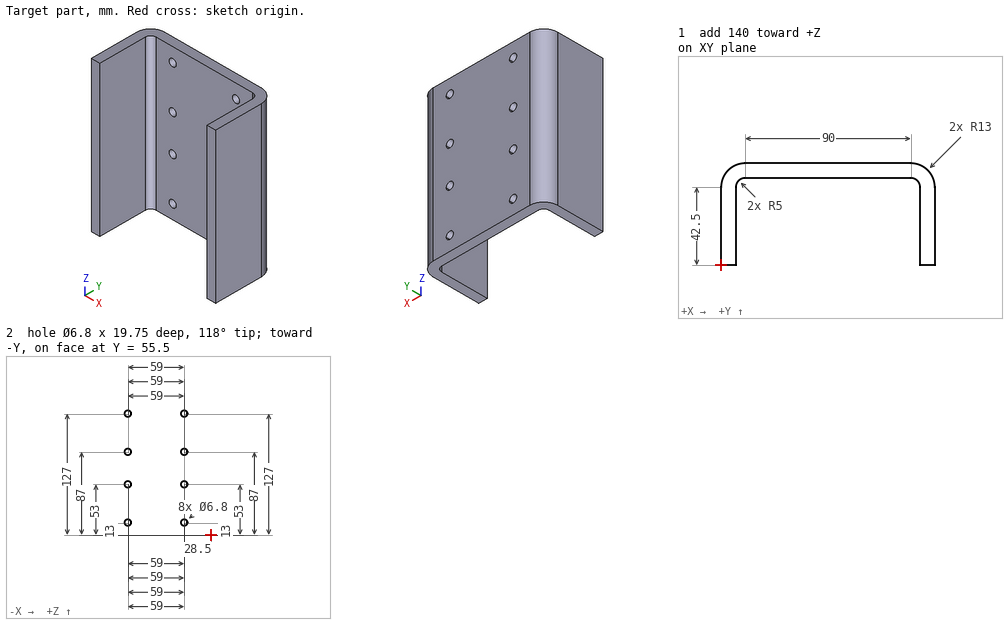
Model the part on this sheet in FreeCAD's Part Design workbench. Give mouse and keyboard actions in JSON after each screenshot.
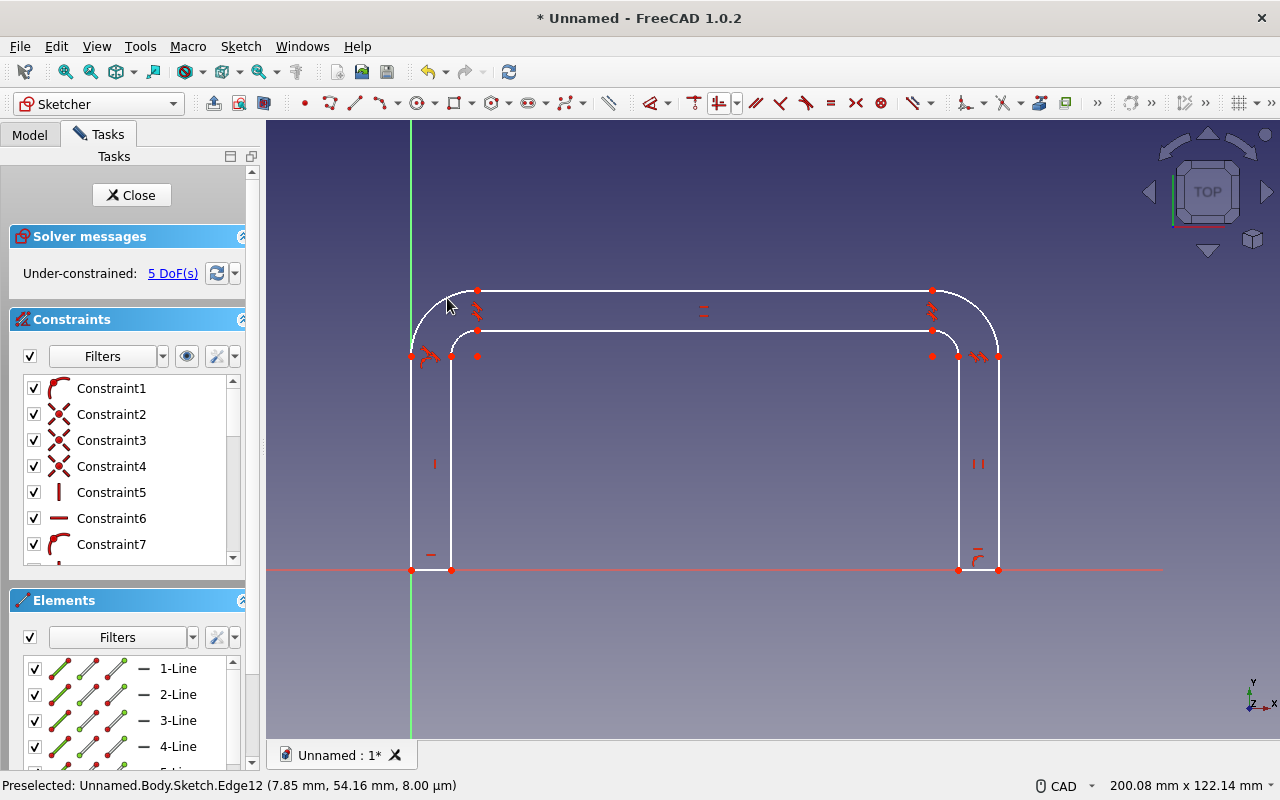
{"action": "left_click", "coordinate": [465, 333]}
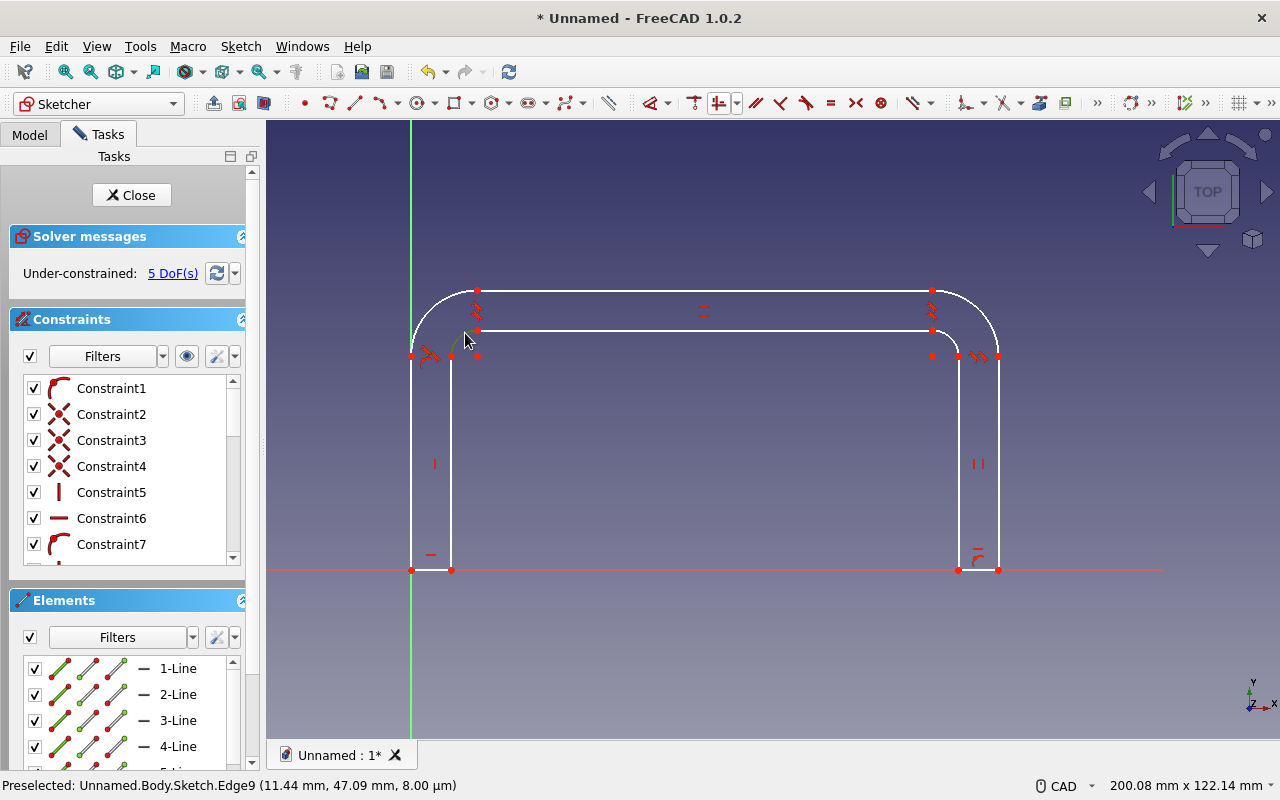
{"action": "left_click", "coordinate": [956, 345]}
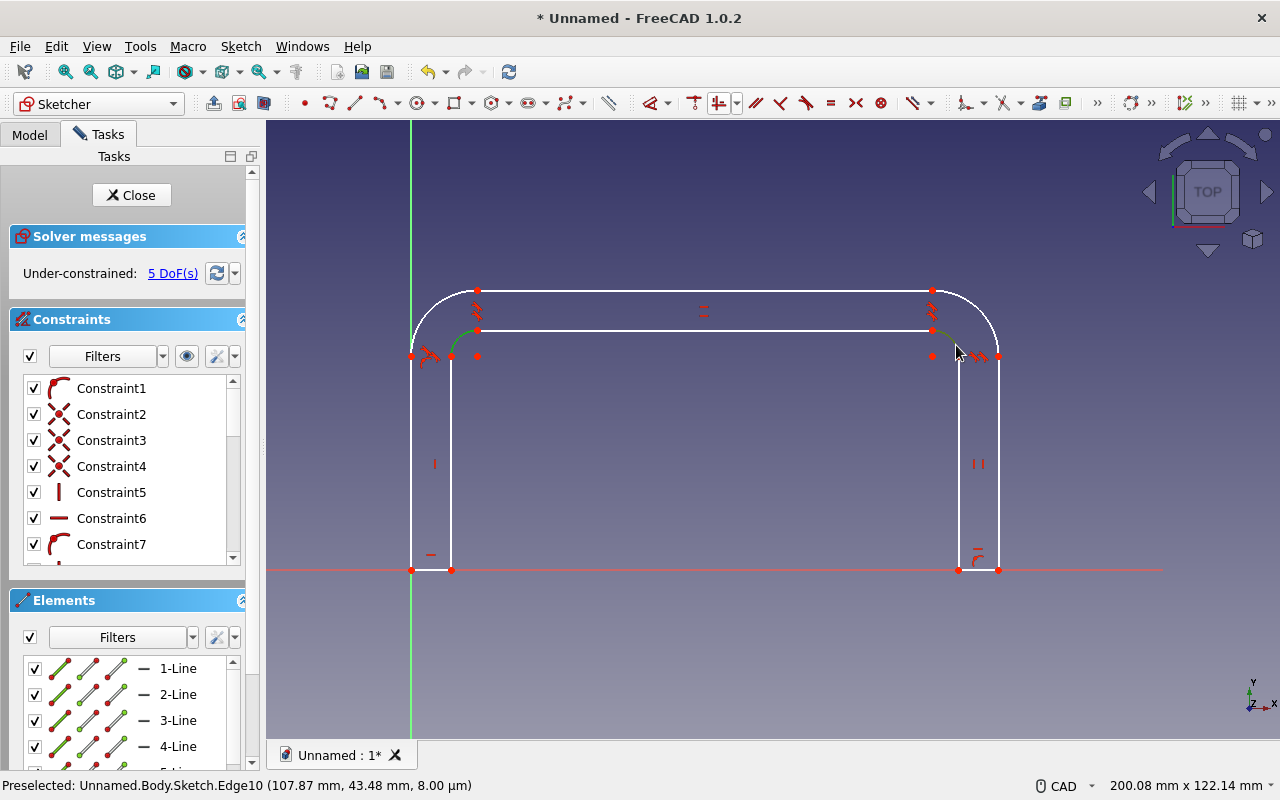
{"action": "left_click", "coordinate": [831, 104]}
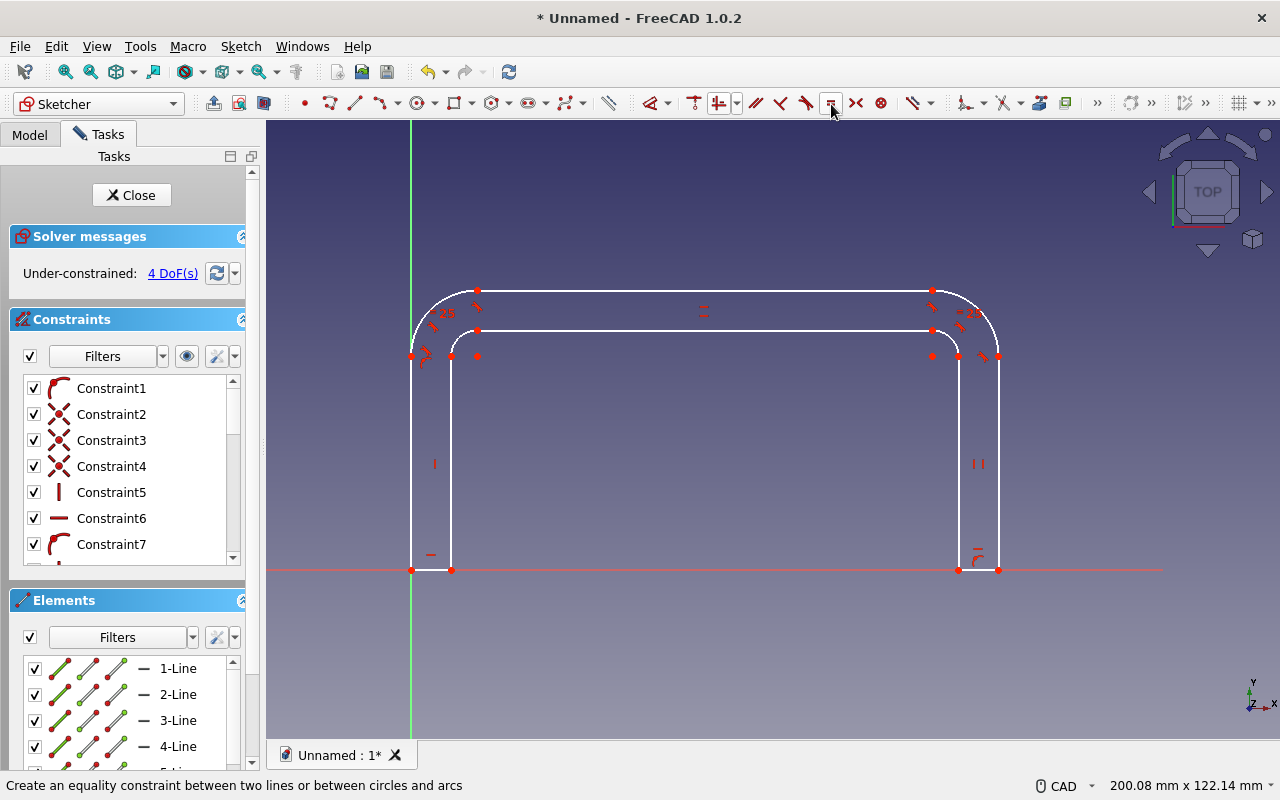
{"action": "key", "text": "d"}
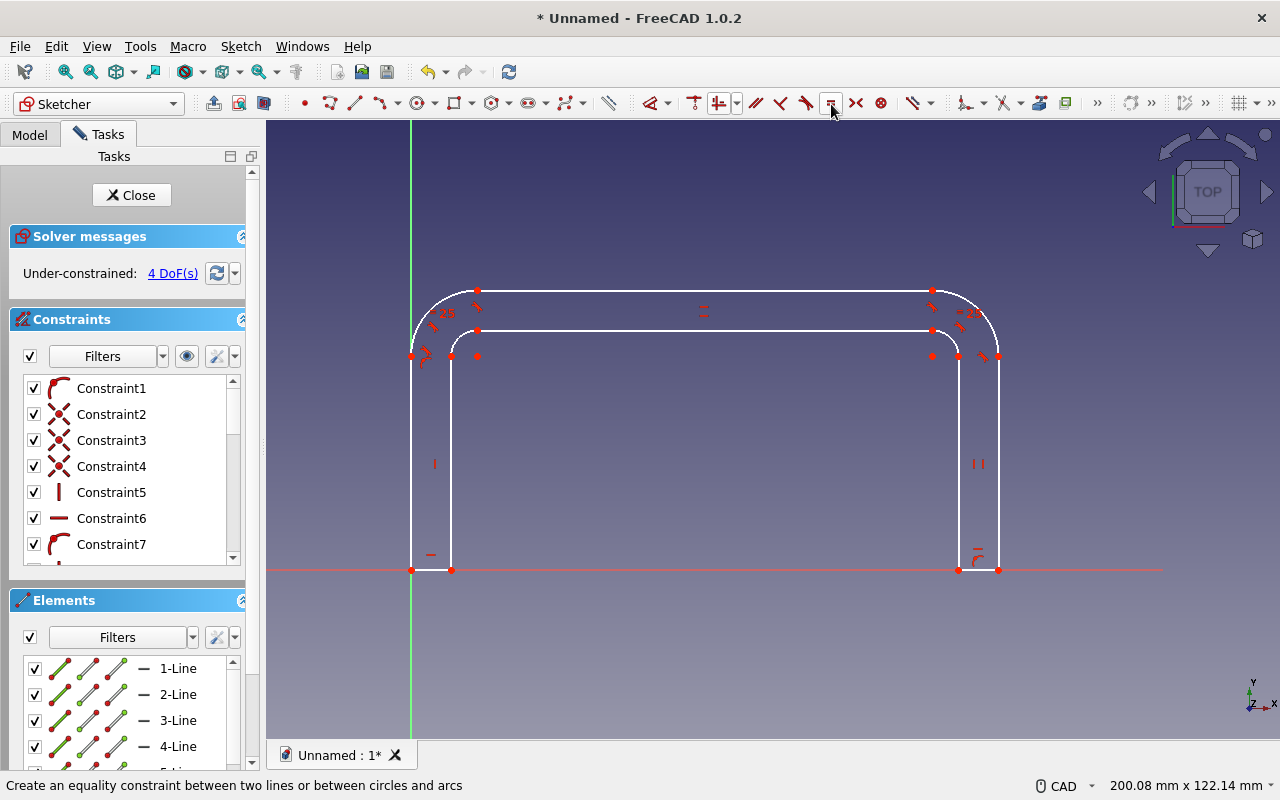
{"action": "scroll", "coordinate": [465, 333], "scroll_direction": "up", "scroll_amount": 3}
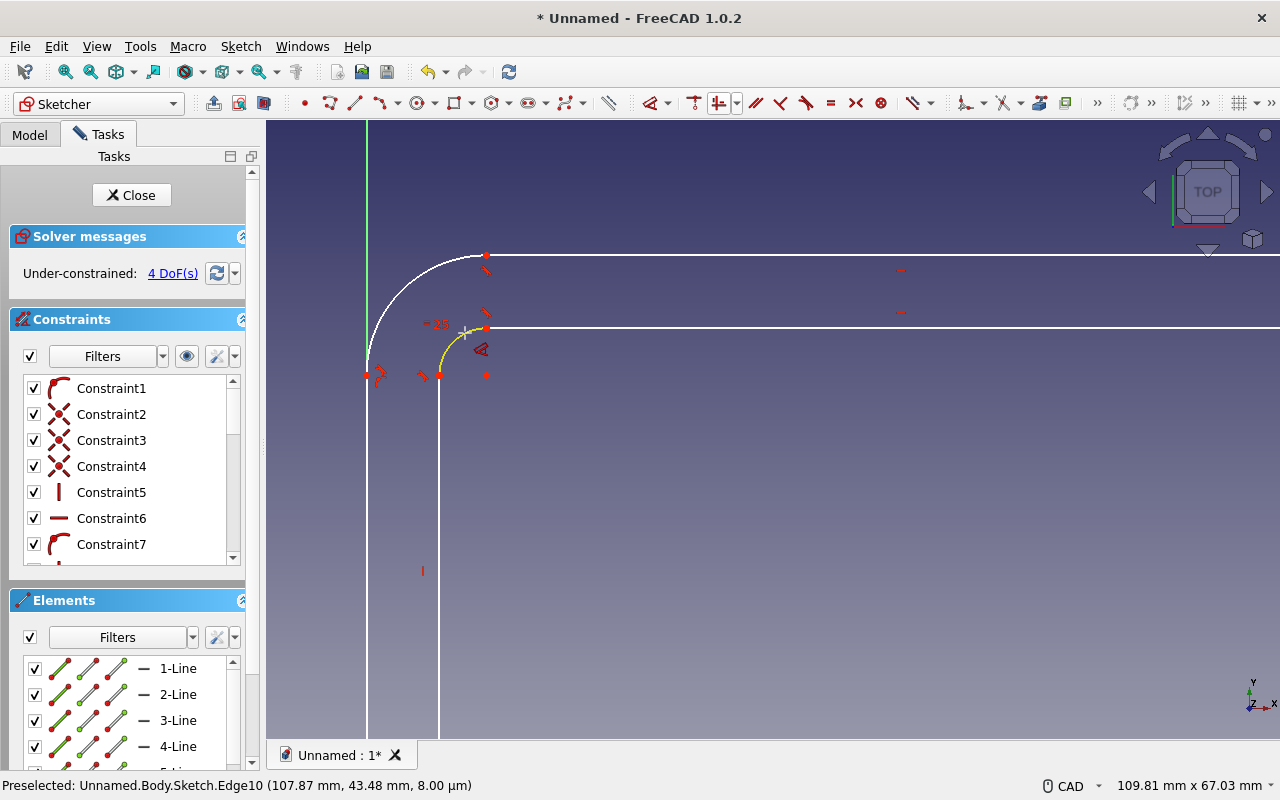
{"action": "left_click", "coordinate": [465, 333]}
{"action": "left_click", "coordinate": [450, 305]}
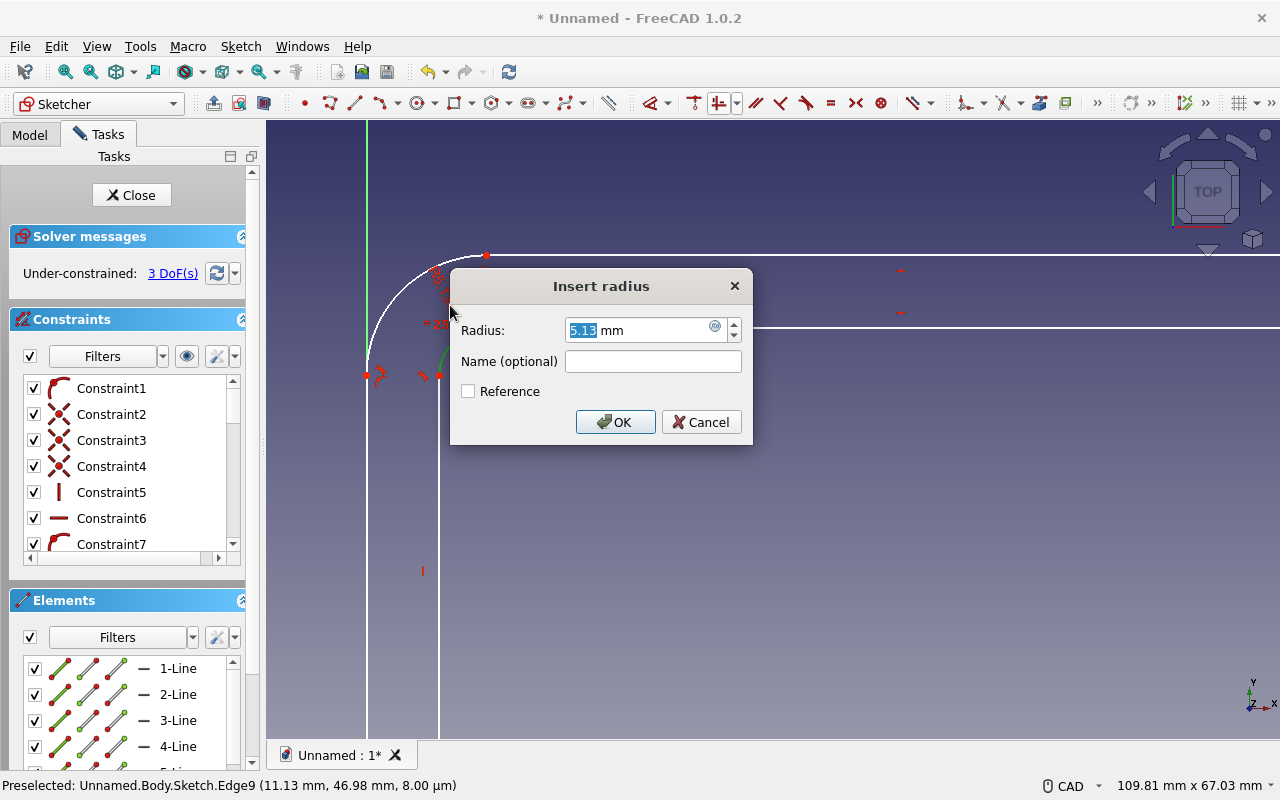
{"action": "type", "text": "5"}
{"action": "key", "text": "Return"}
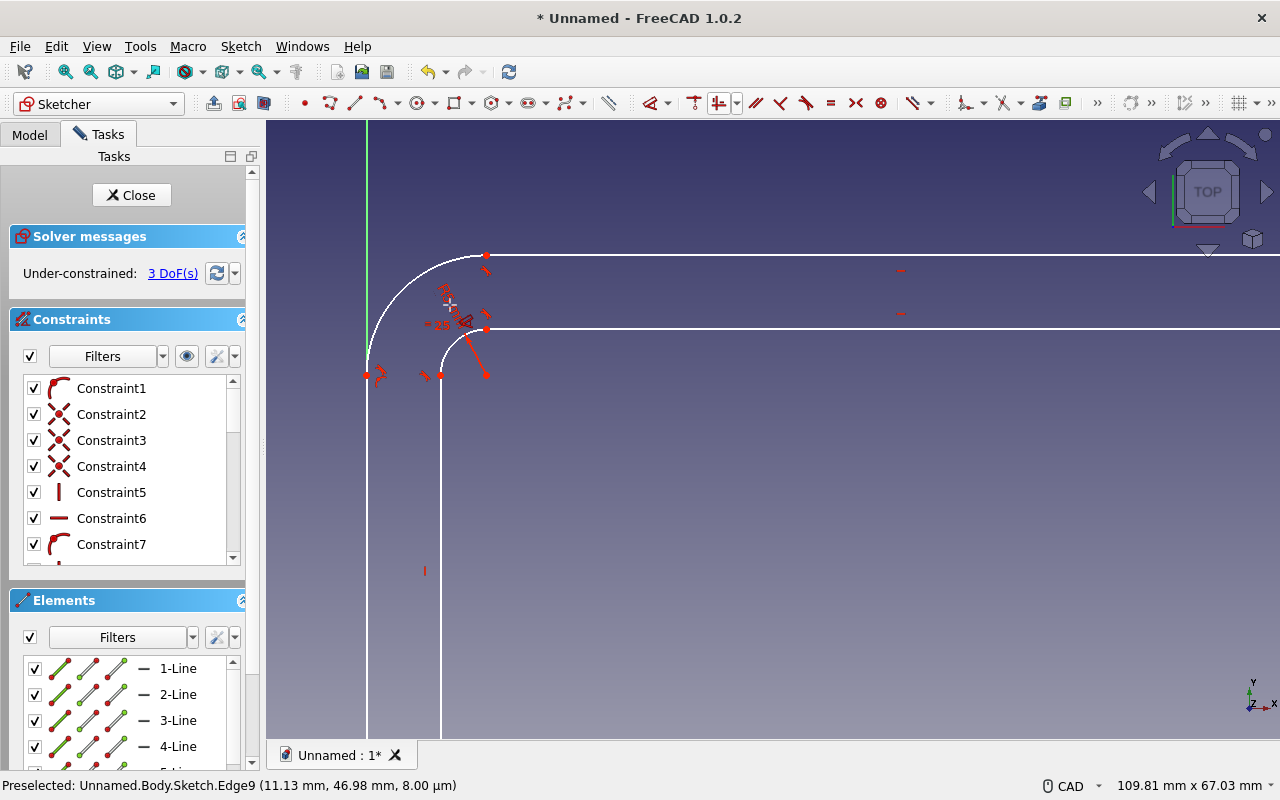
{"action": "scroll", "coordinate": [464, 333], "scroll_direction": "down", "scroll_amount": 3}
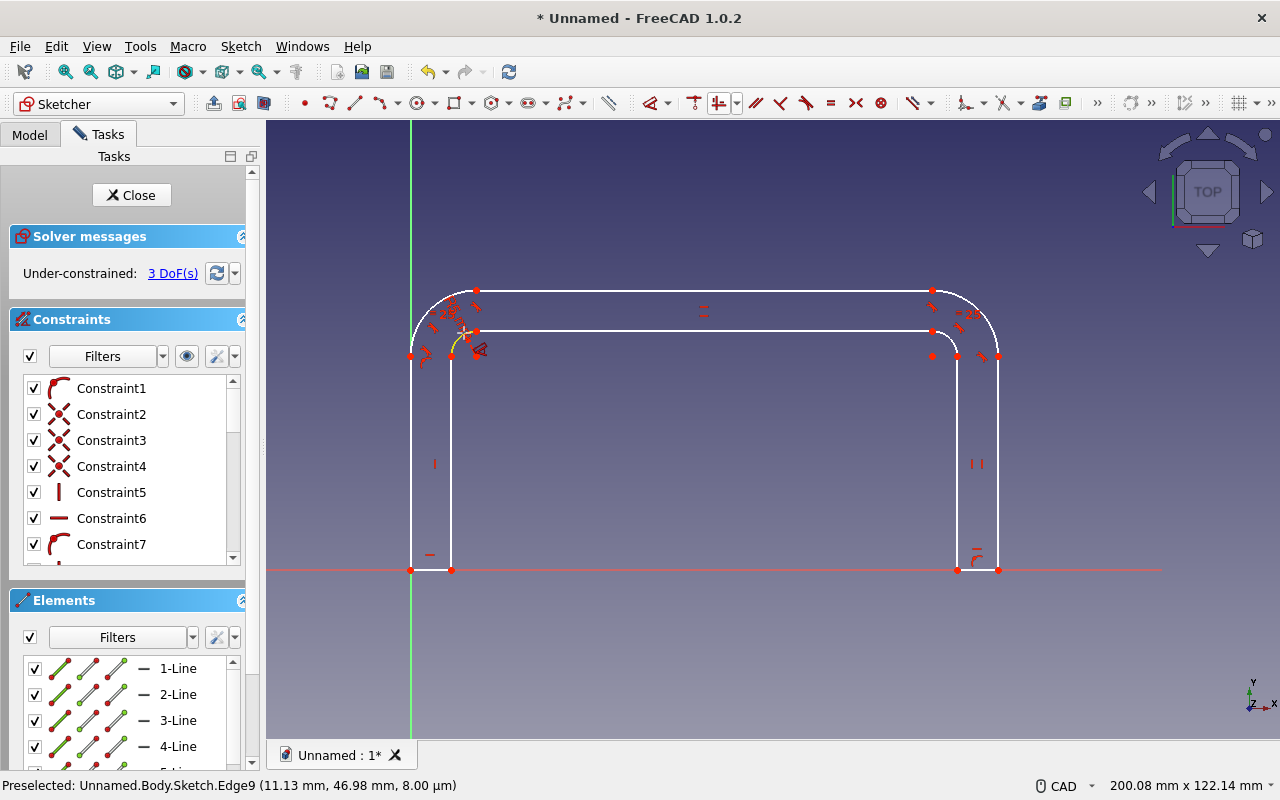
{"action": "left_click", "coordinate": [991, 327]}
{"action": "left_click", "coordinate": [1020, 313]}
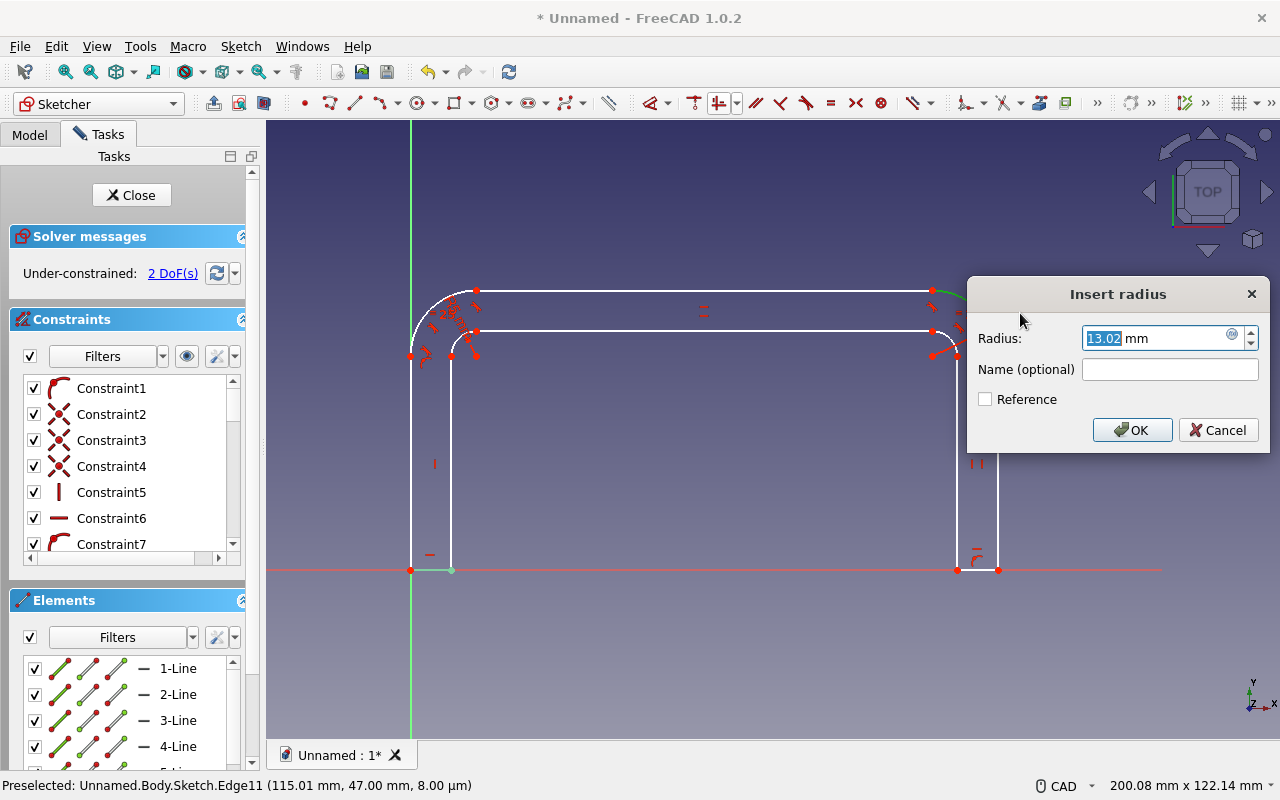
{"action": "type", "text": "13"}
{"action": "key", "text": "Return"}